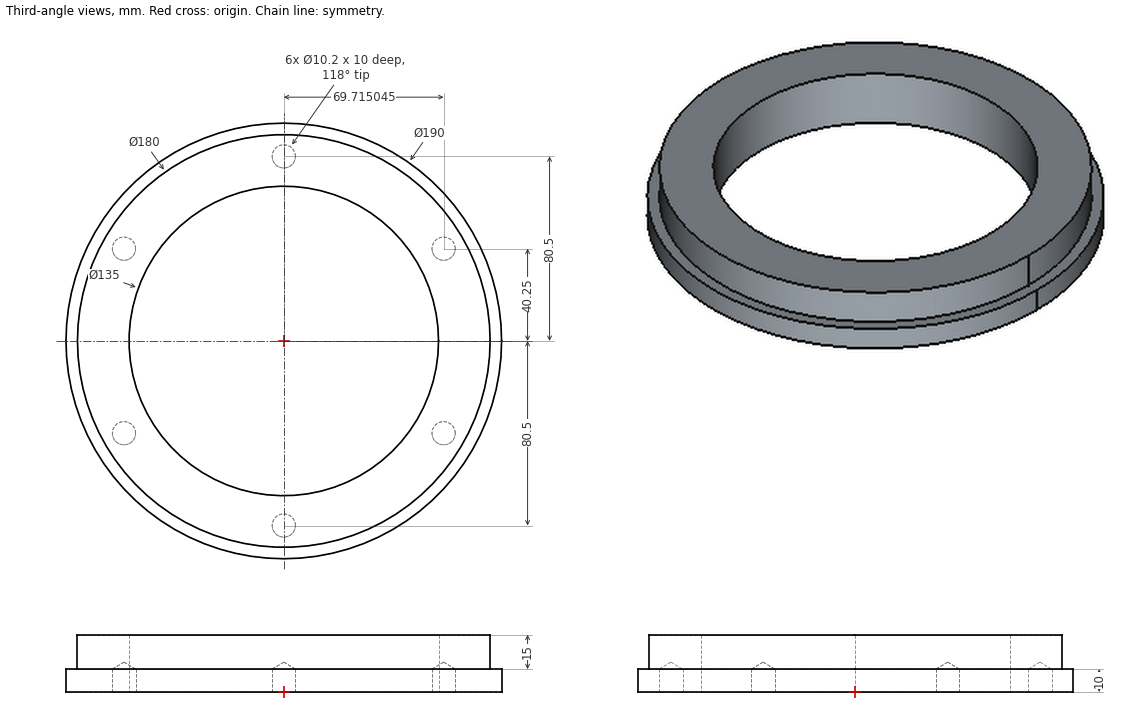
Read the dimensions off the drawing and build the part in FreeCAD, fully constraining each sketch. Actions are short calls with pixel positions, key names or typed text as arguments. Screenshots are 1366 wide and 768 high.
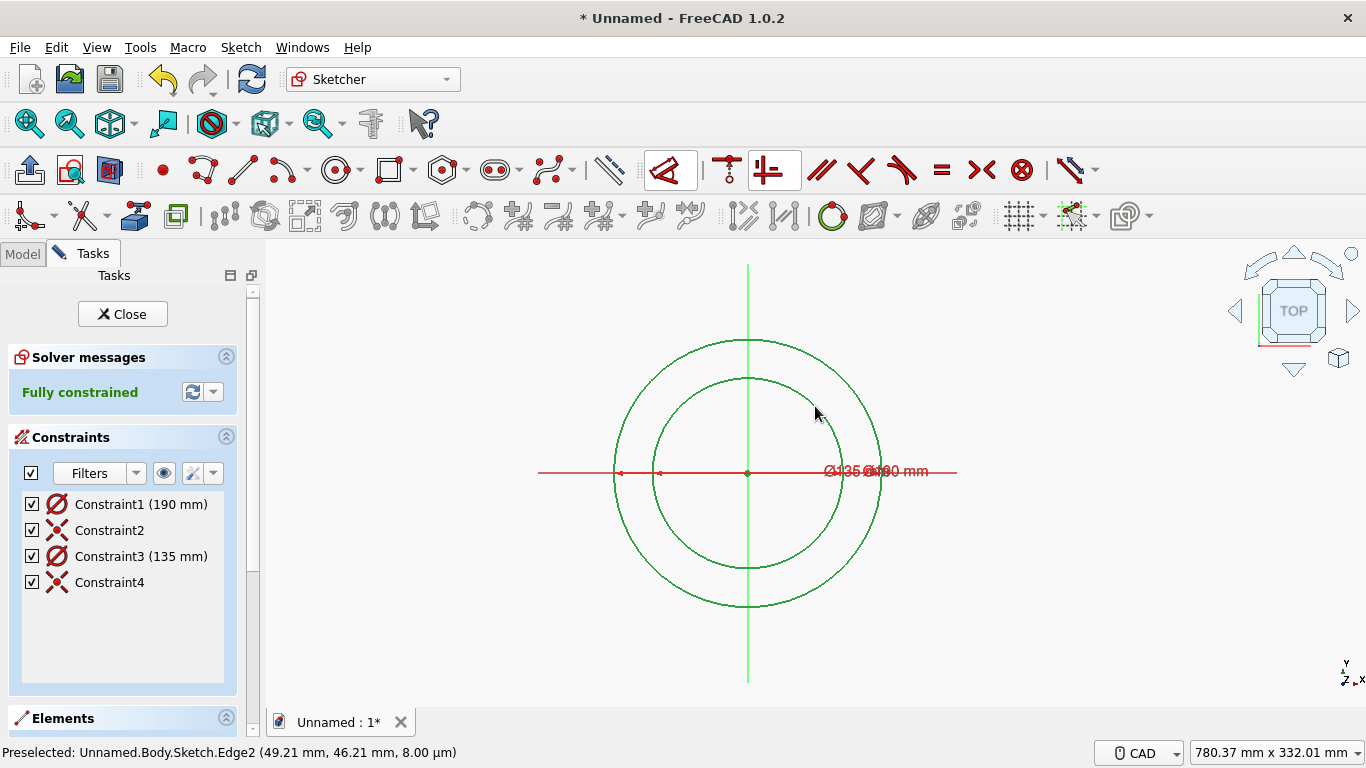
click(123, 314)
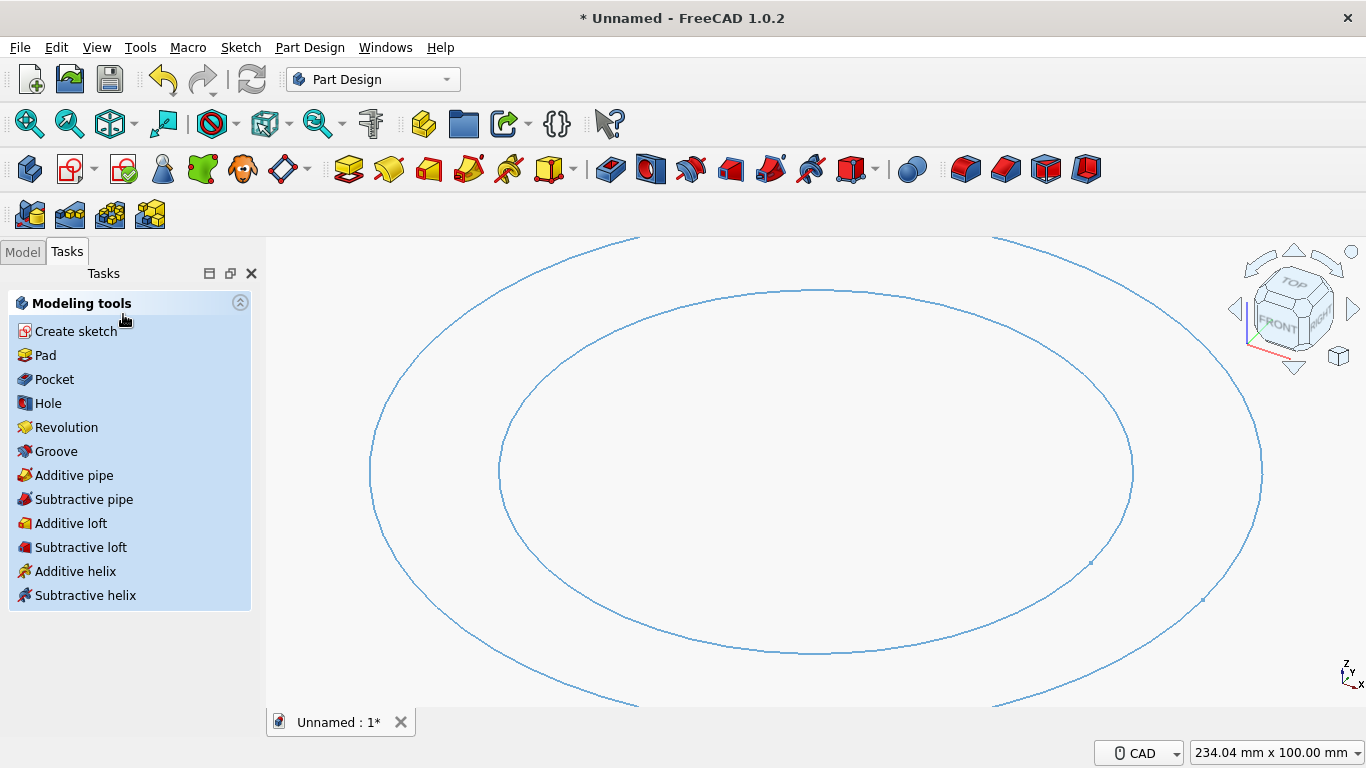
click(350, 170)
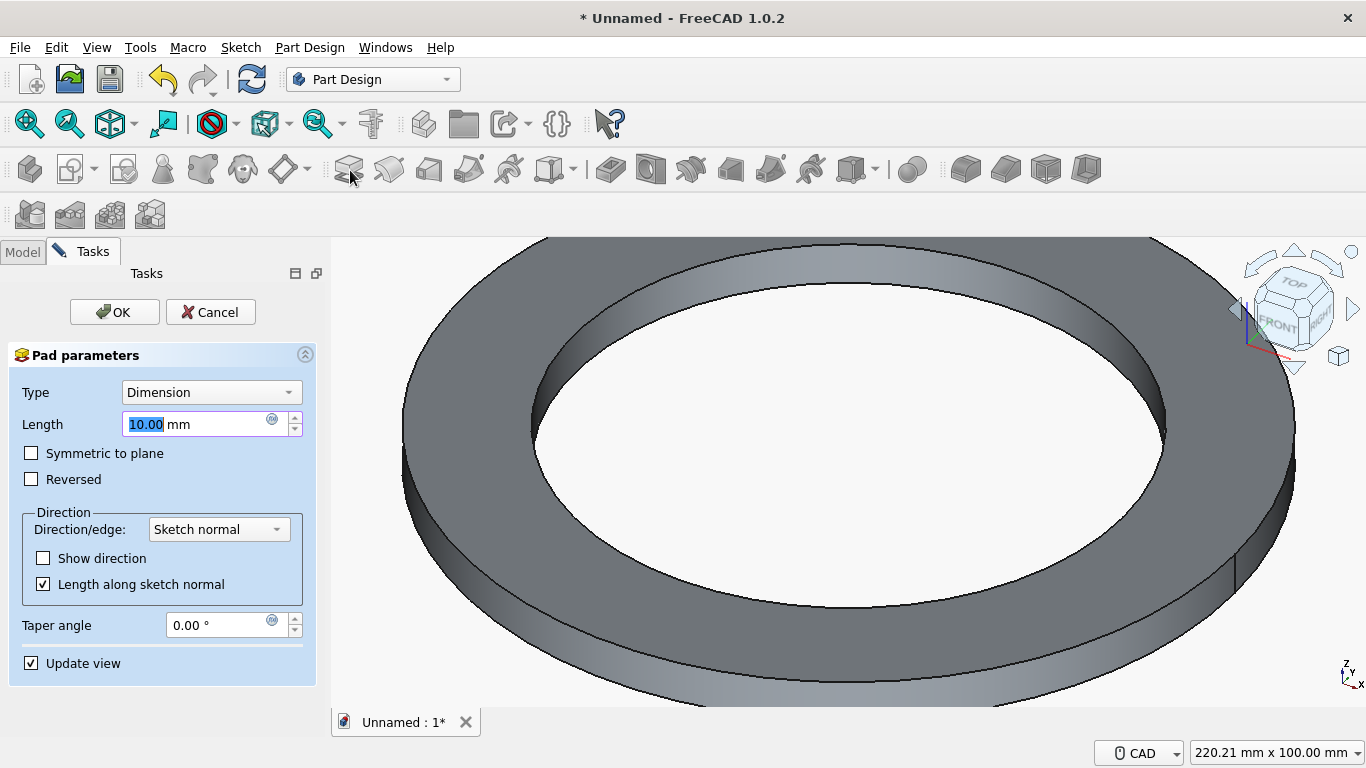
text(10)
key(Tab)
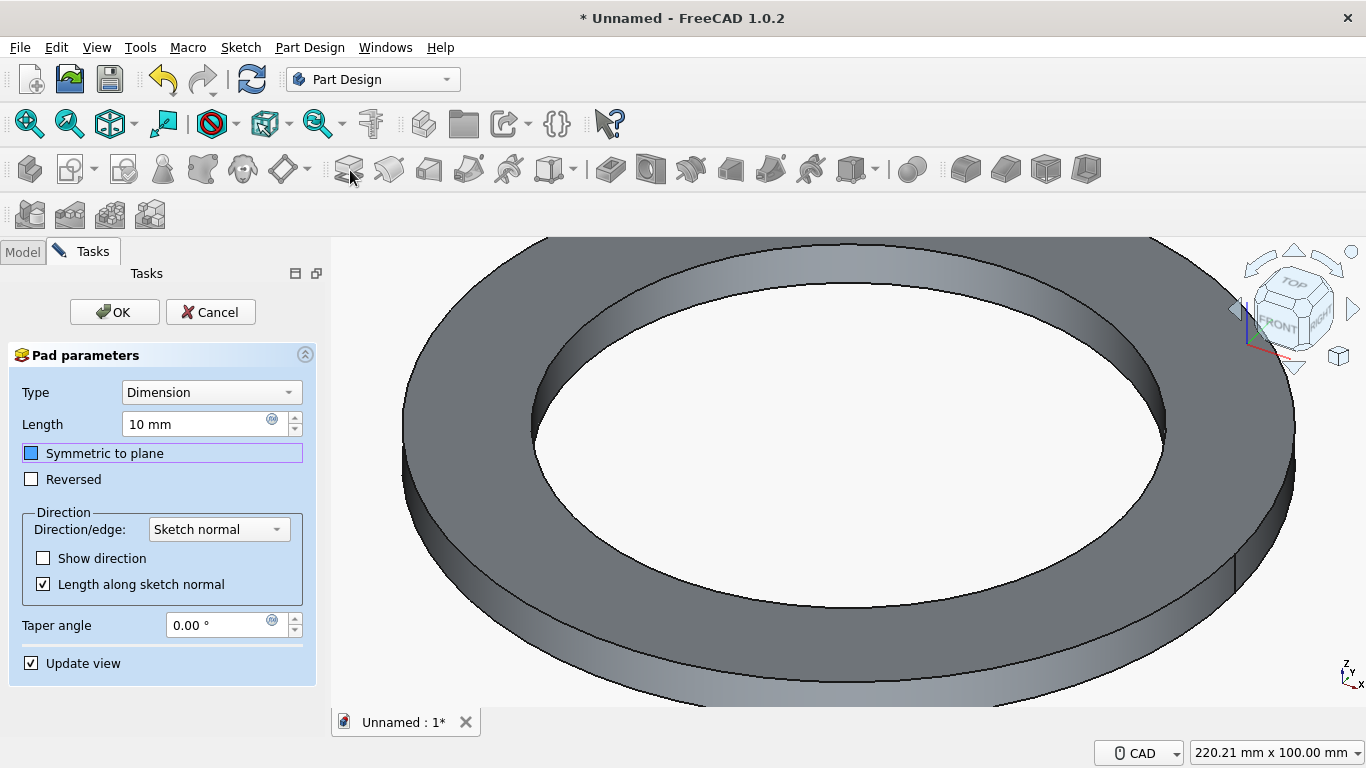
click(115, 312)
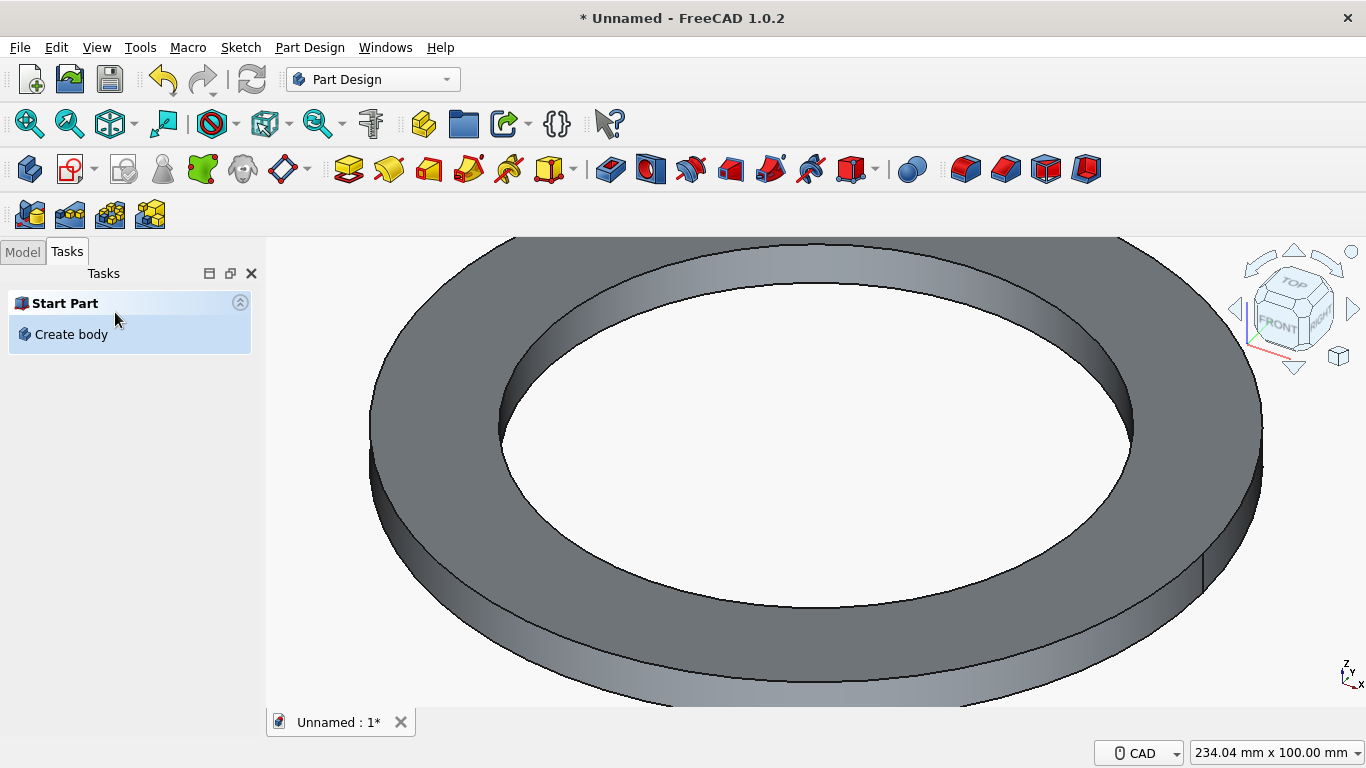
key(v)
key(f)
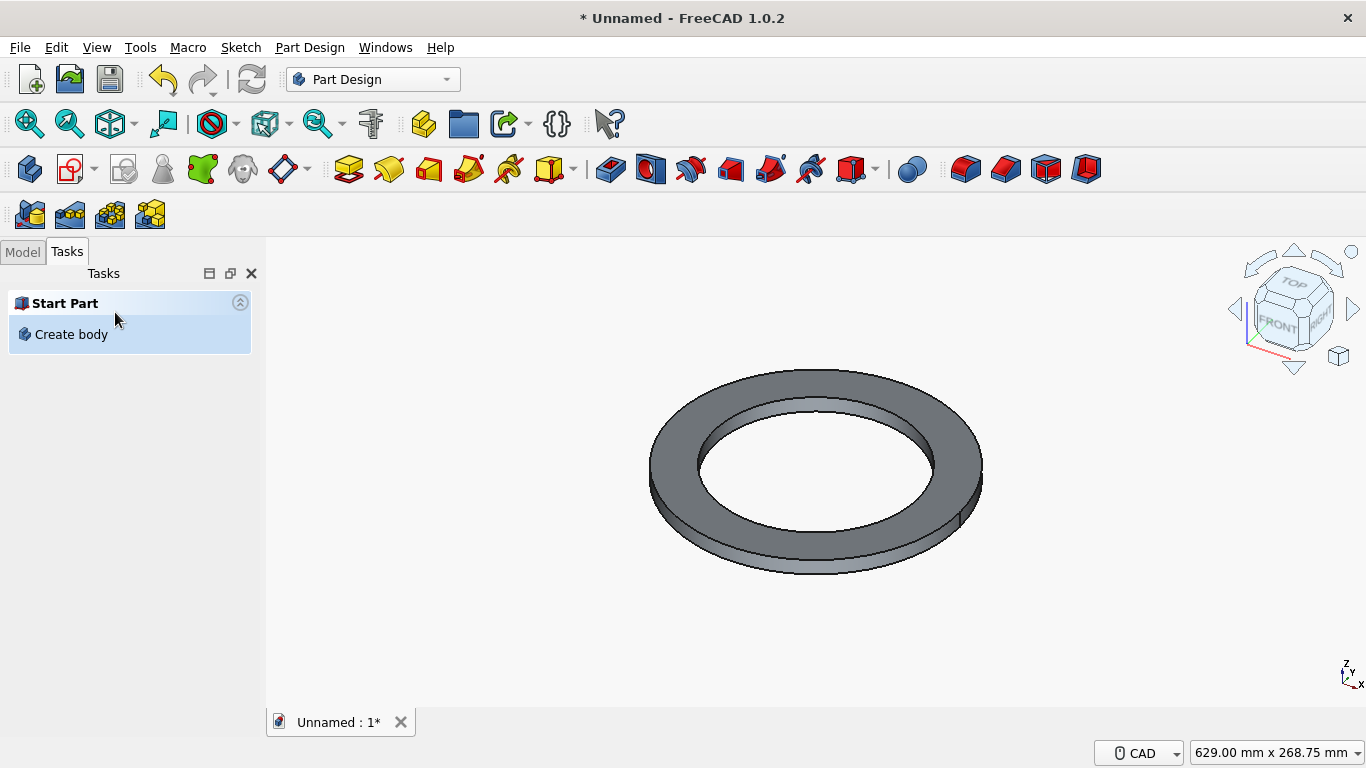
click(939, 505)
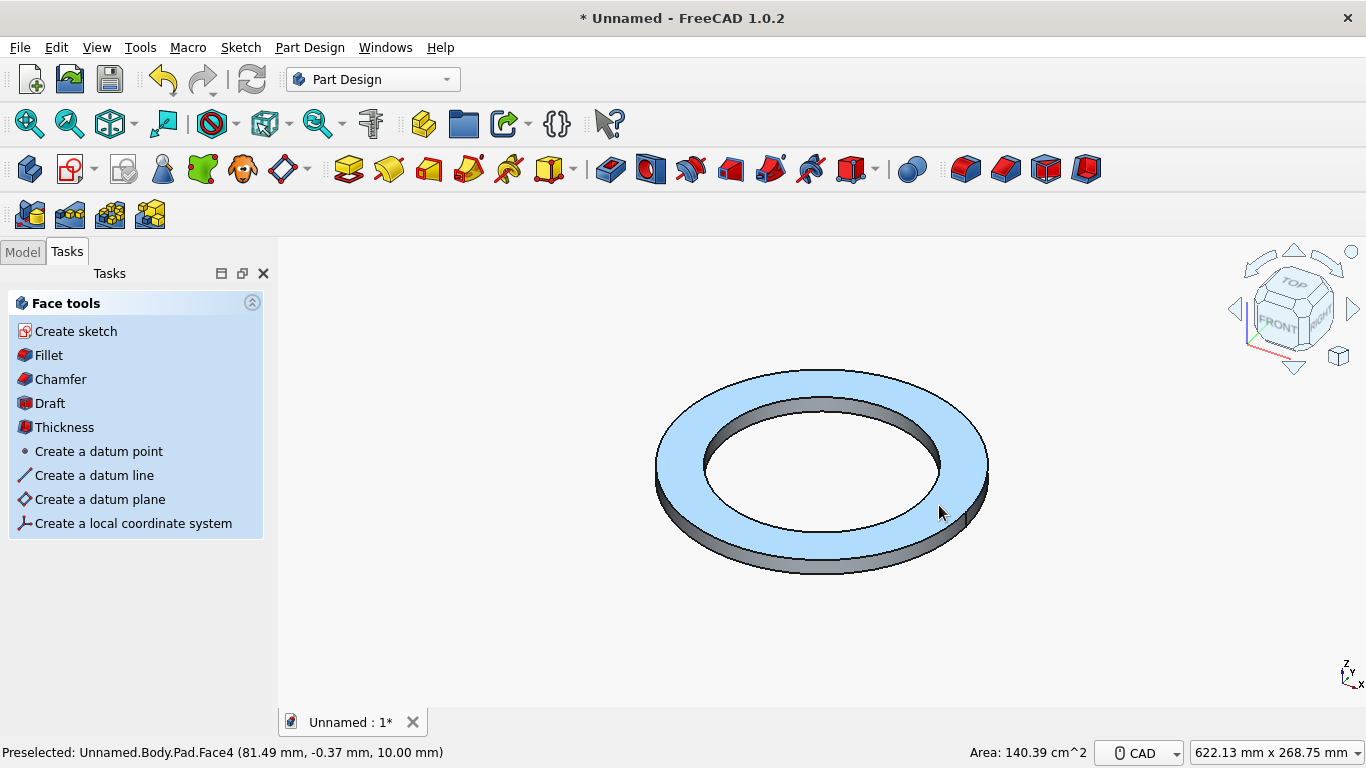
click(70, 170)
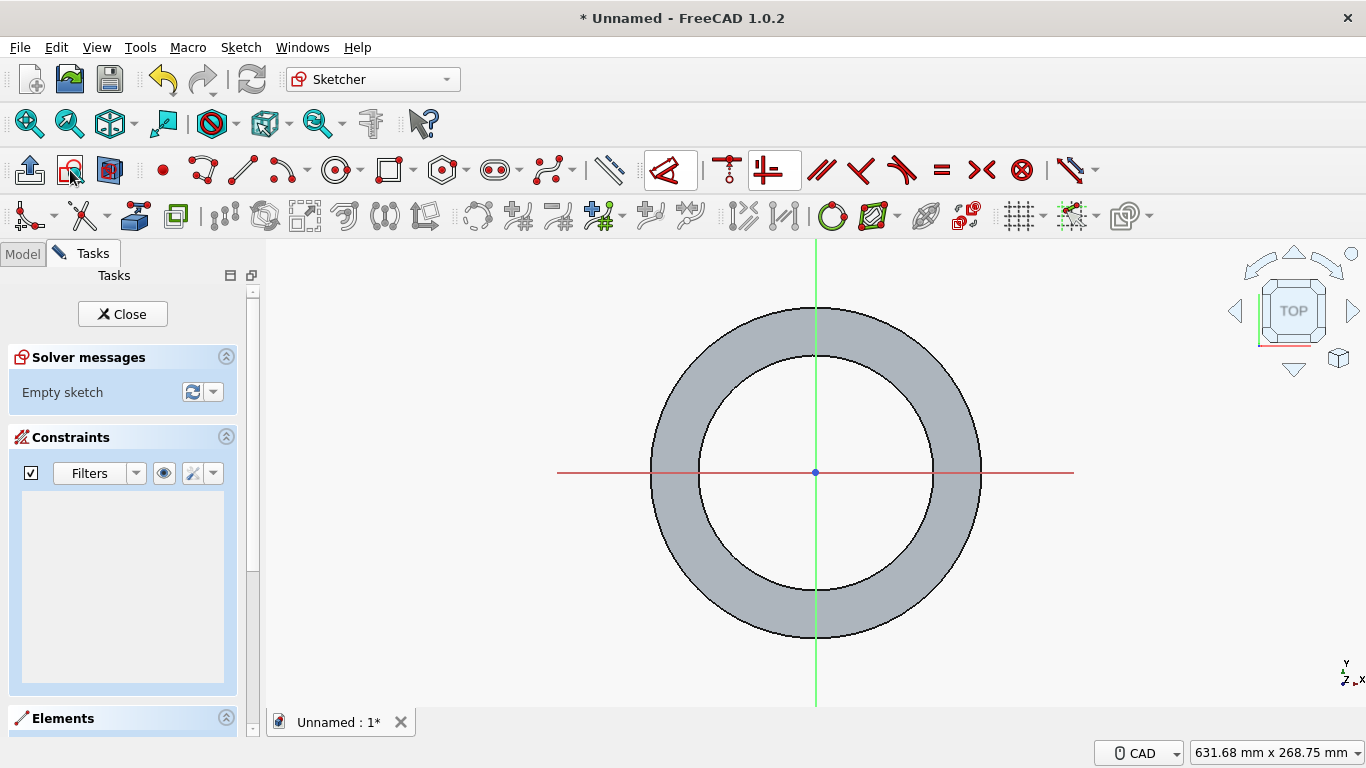
key(g)
key(c)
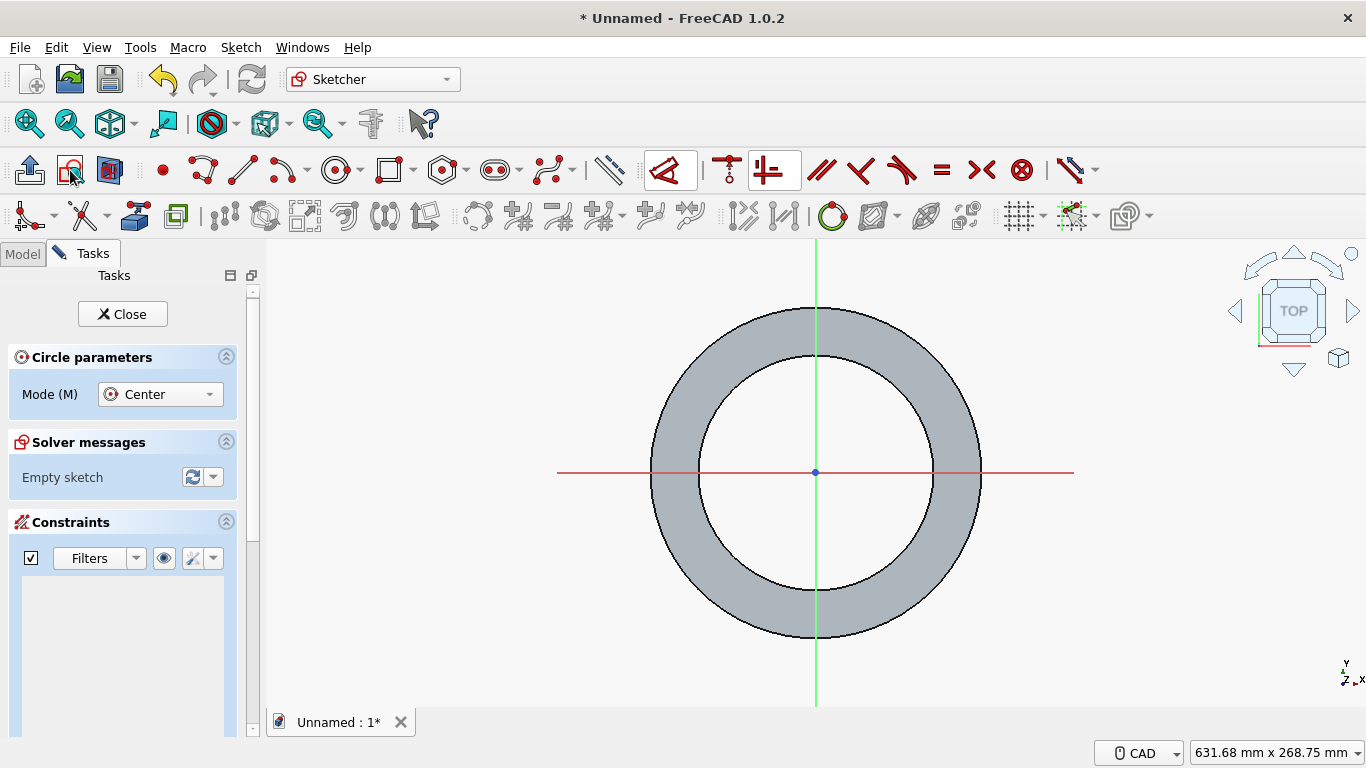
click(816, 473)
move(927, 362)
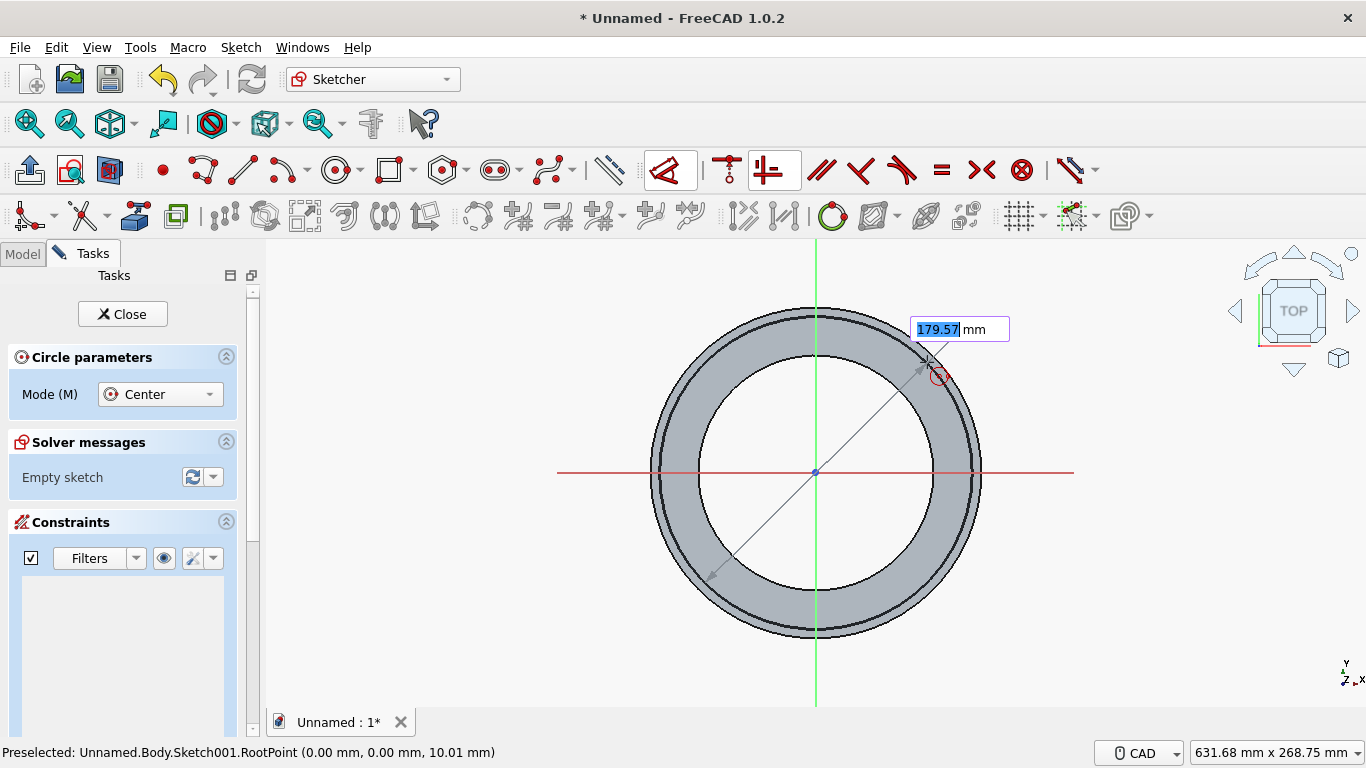
text(180)
key(Return)